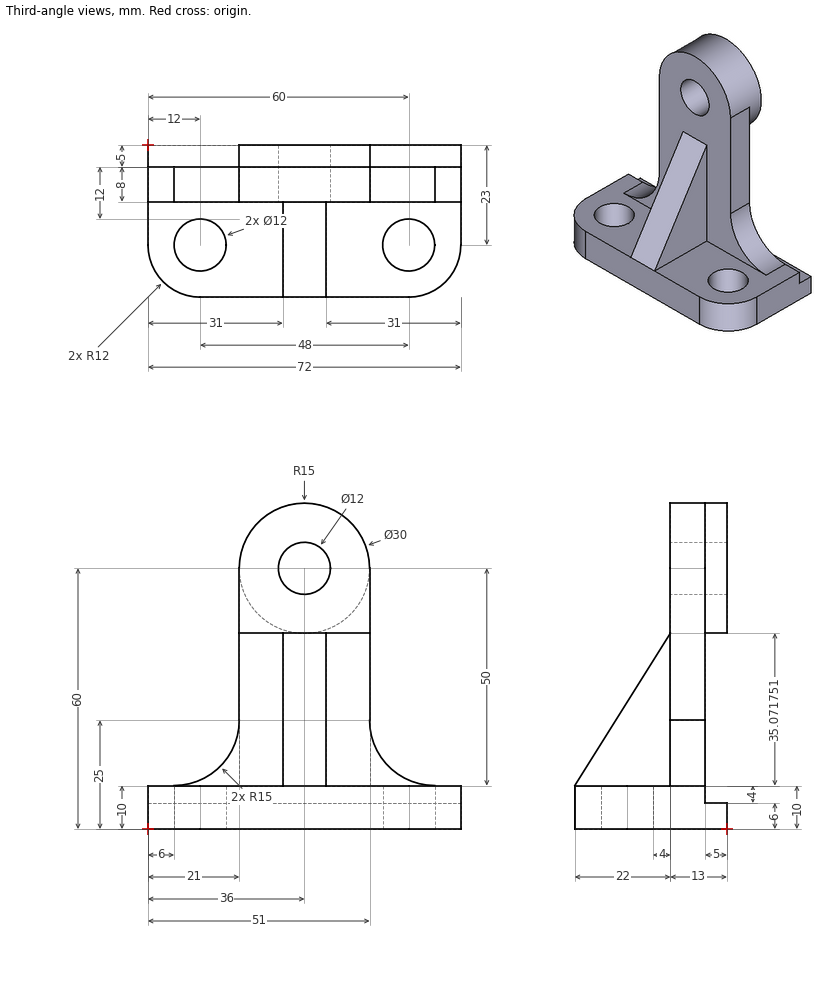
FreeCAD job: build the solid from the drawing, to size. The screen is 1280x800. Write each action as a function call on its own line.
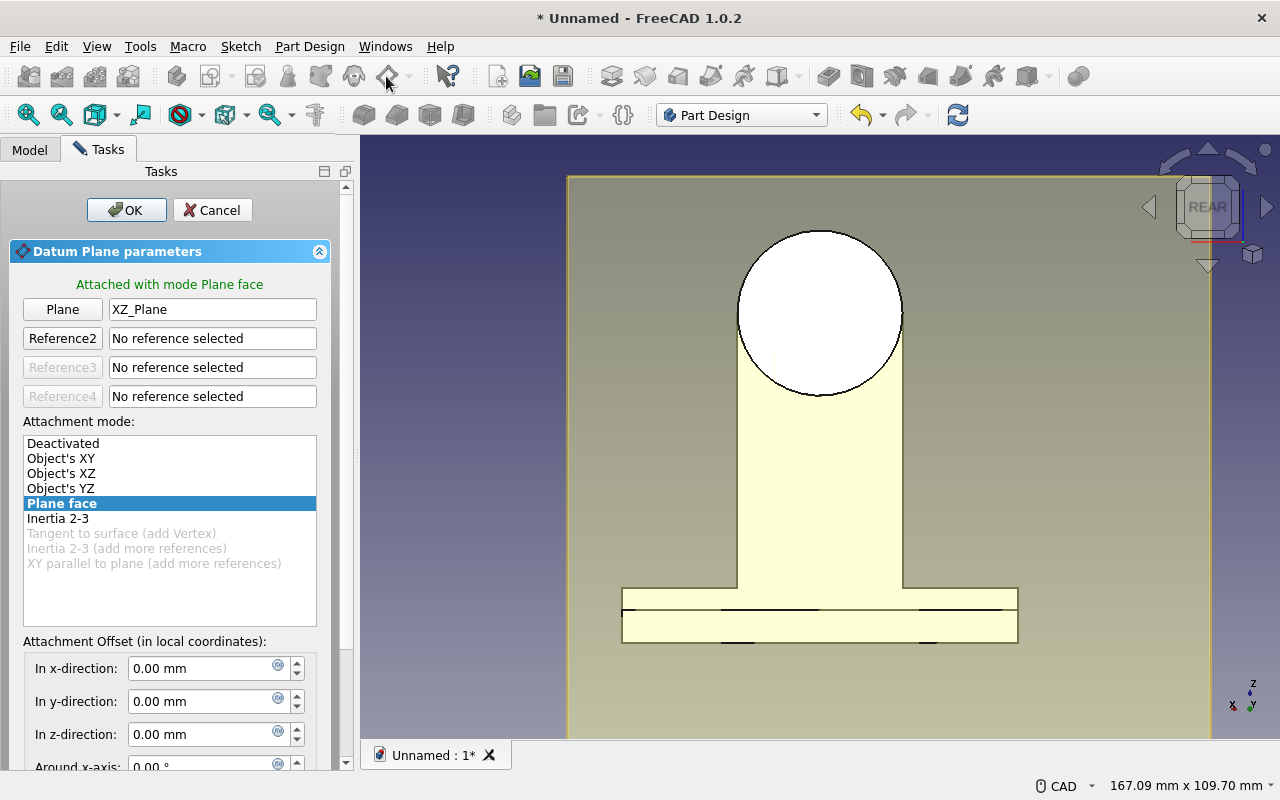
triple_click(210, 734)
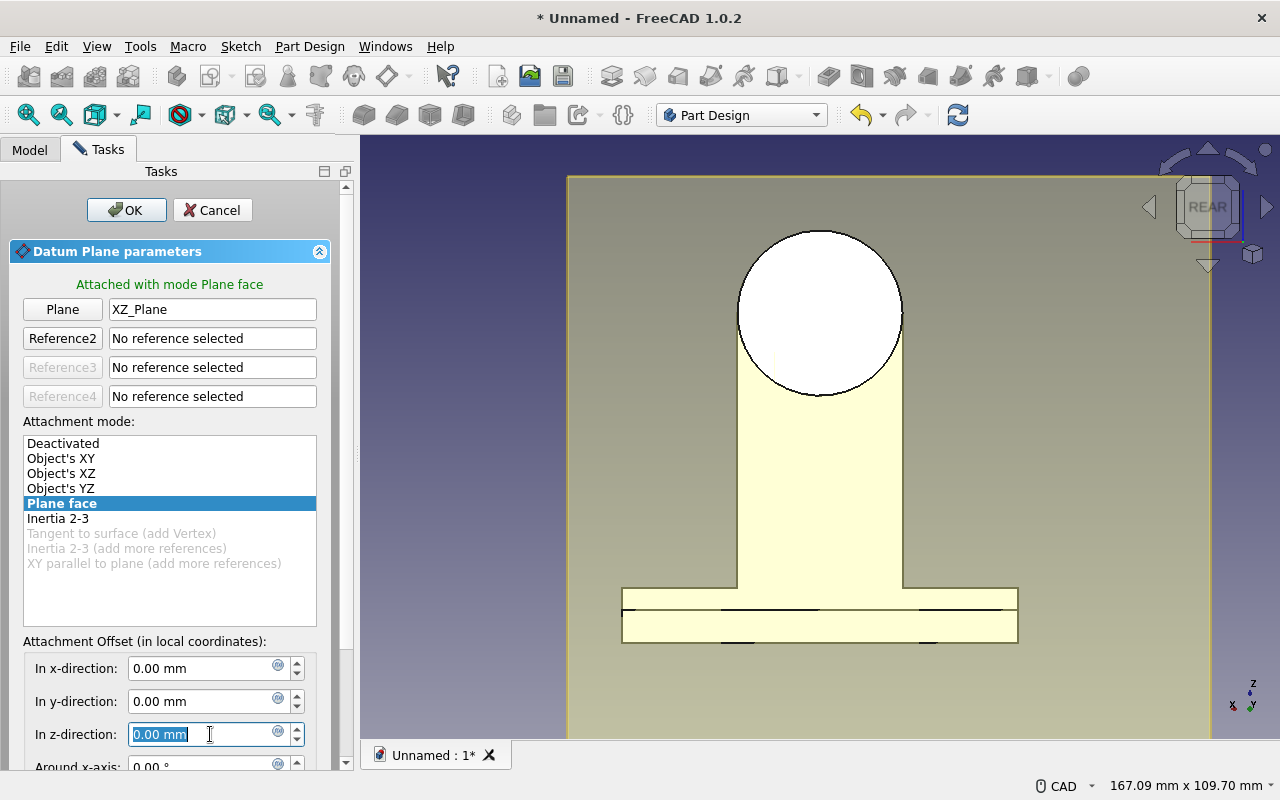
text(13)
key(Tab)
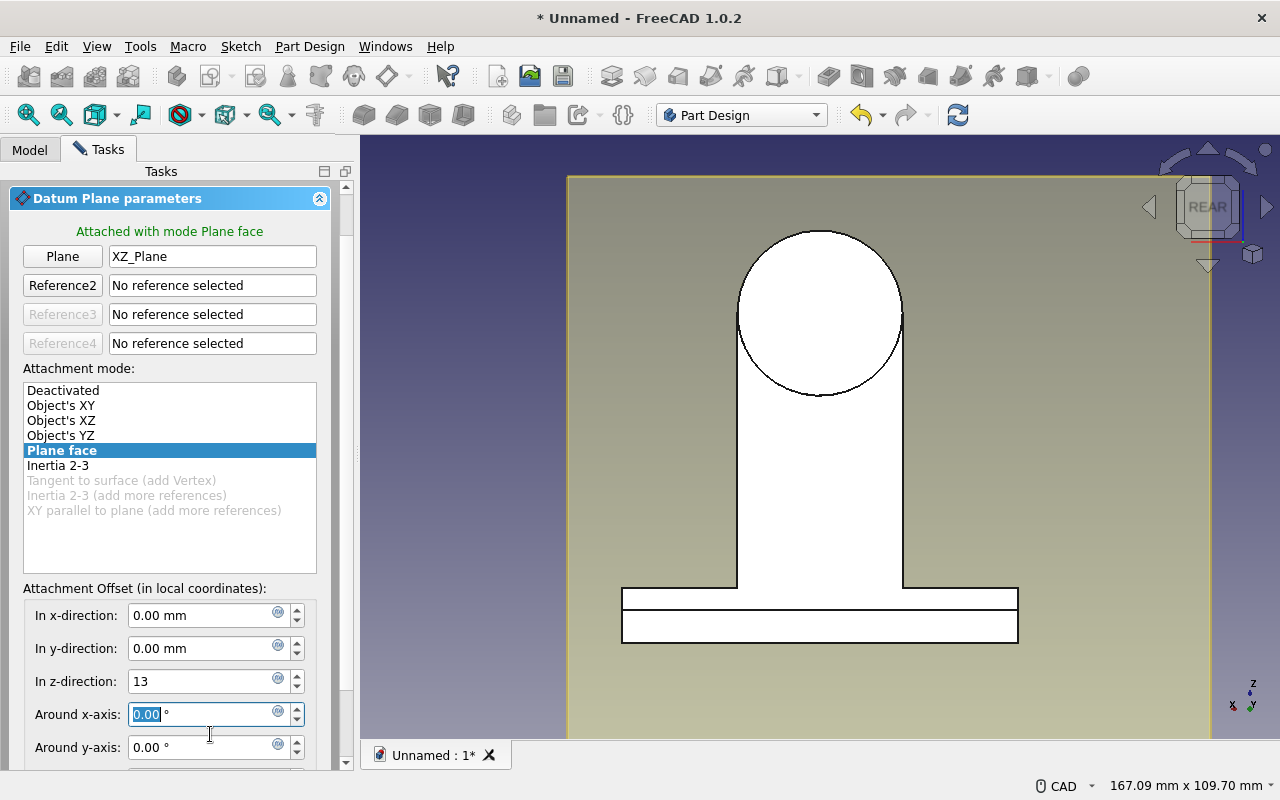
scroll(346, 476, up, 2)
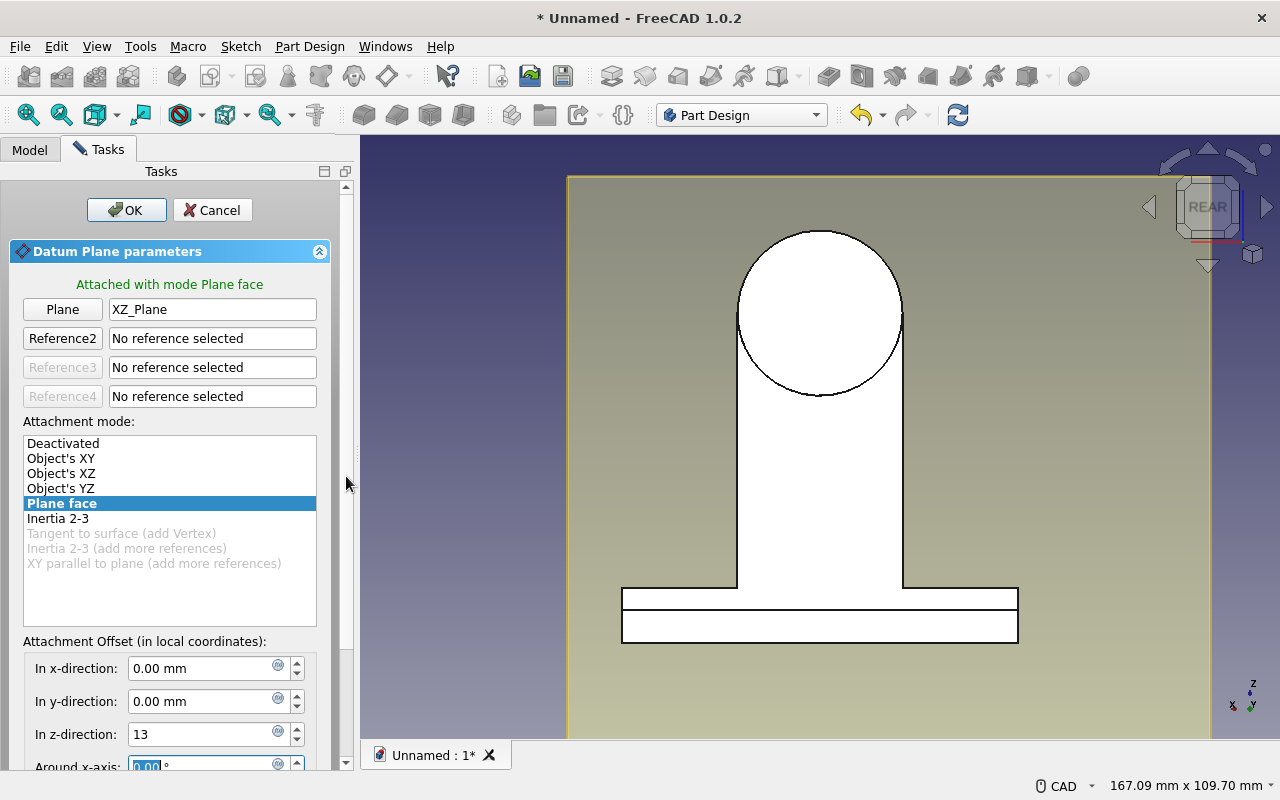
click(127, 210)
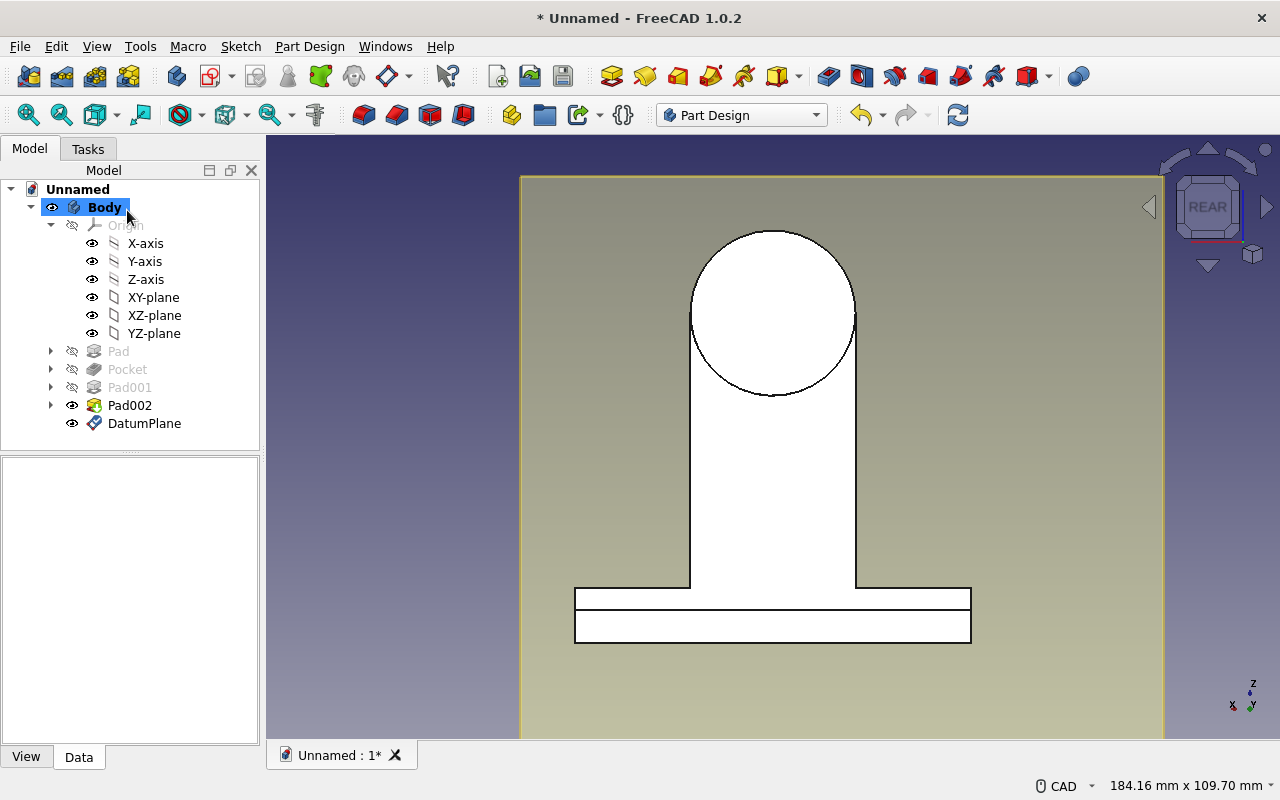
click(117, 423)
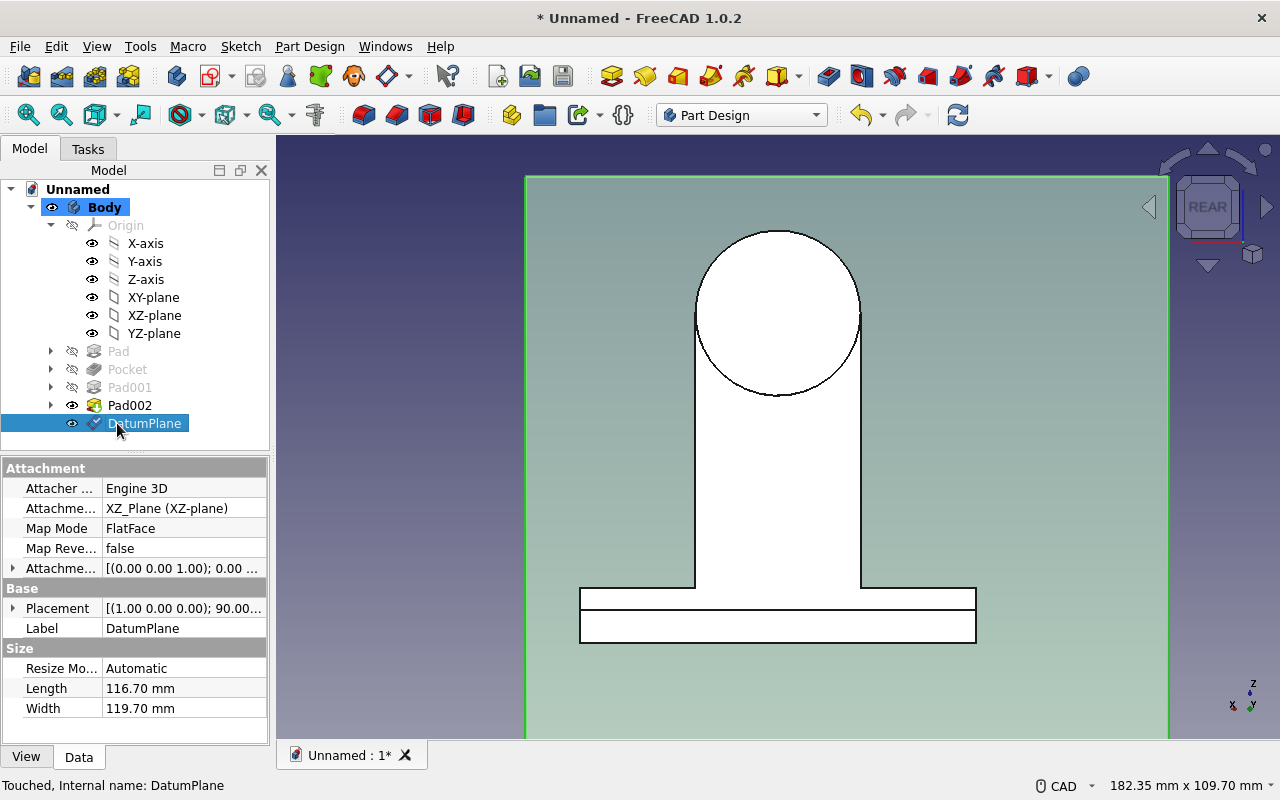
click(210, 76)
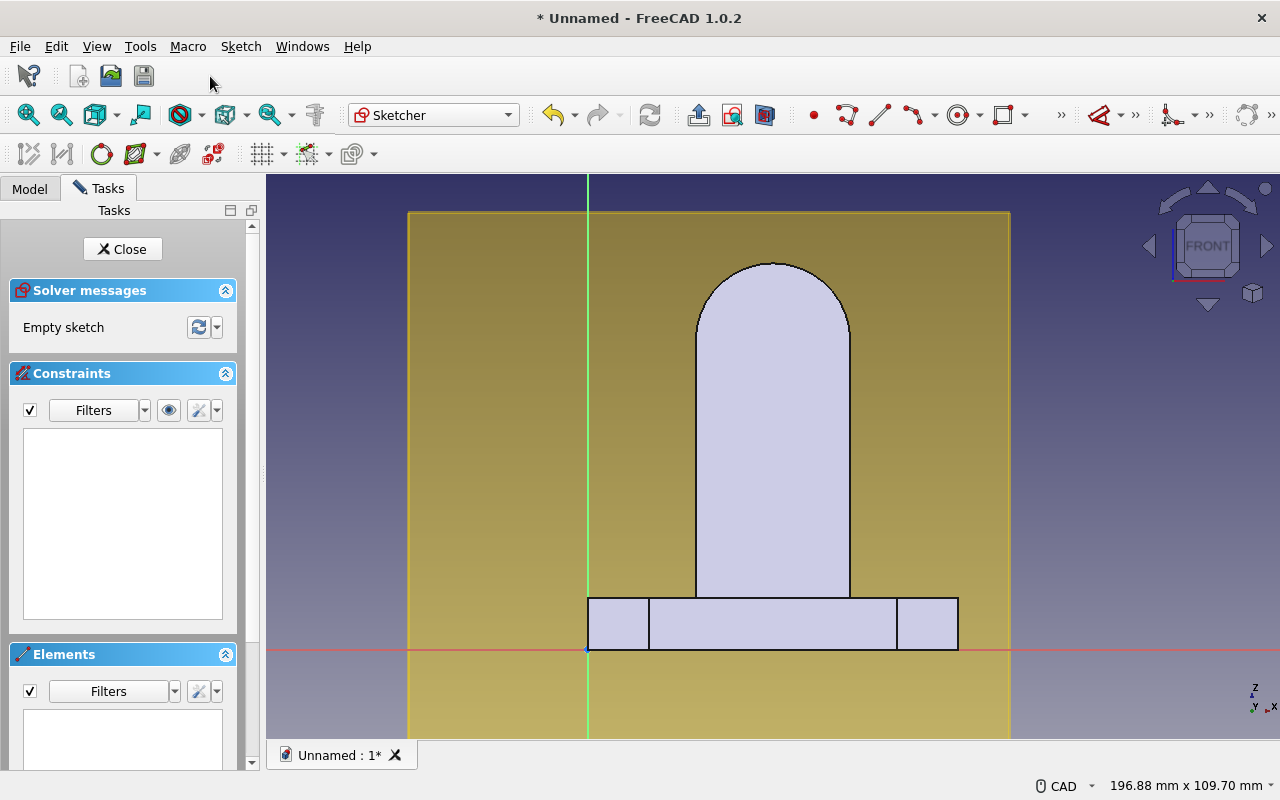
click(765, 116)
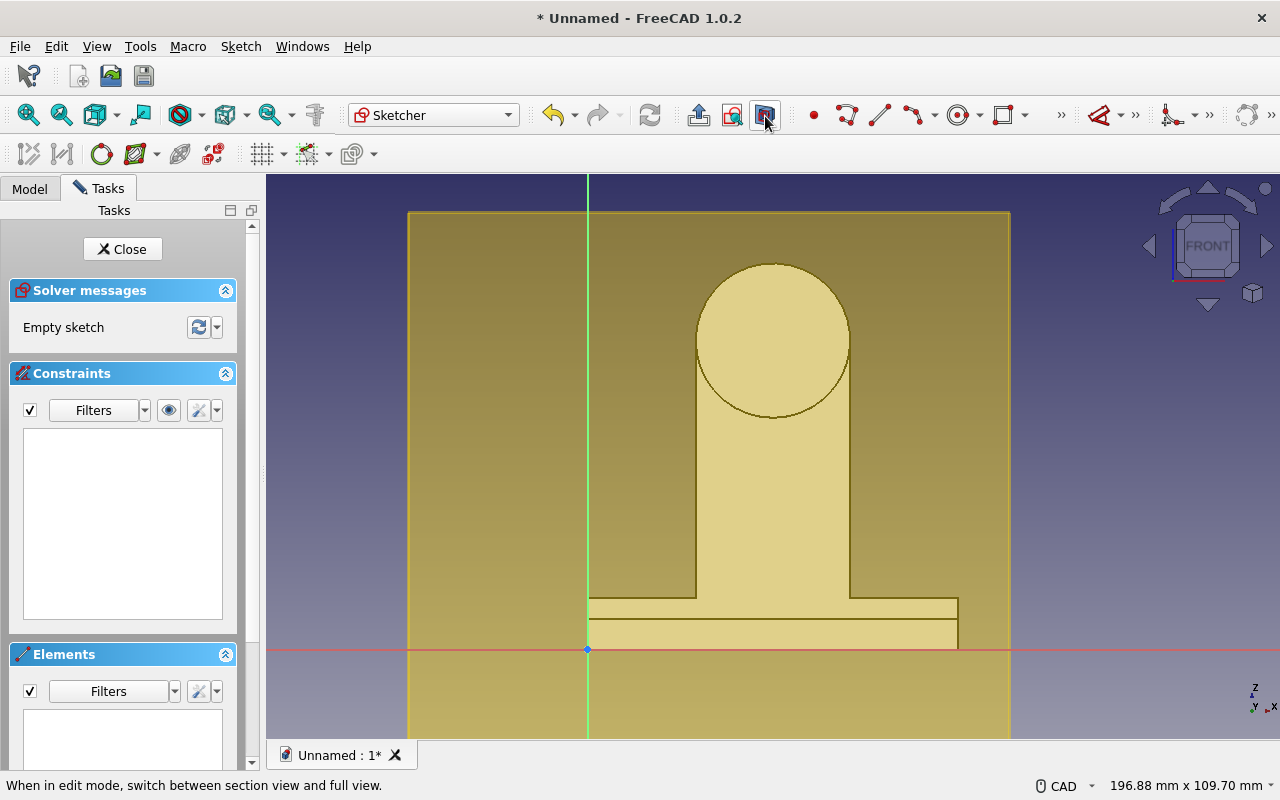
click(847, 116)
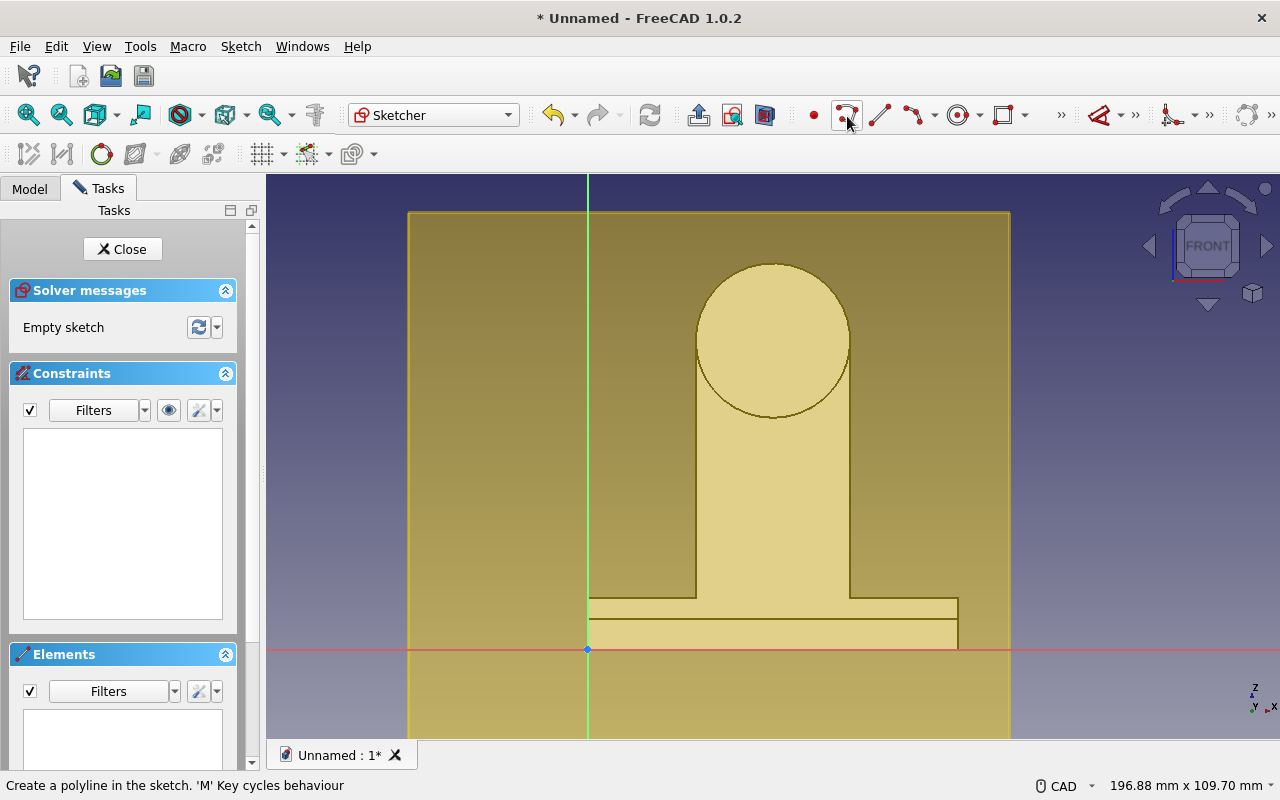
click(696, 341)
click(696, 598)
click(850, 598)
click(850, 341)
right_click(850, 341)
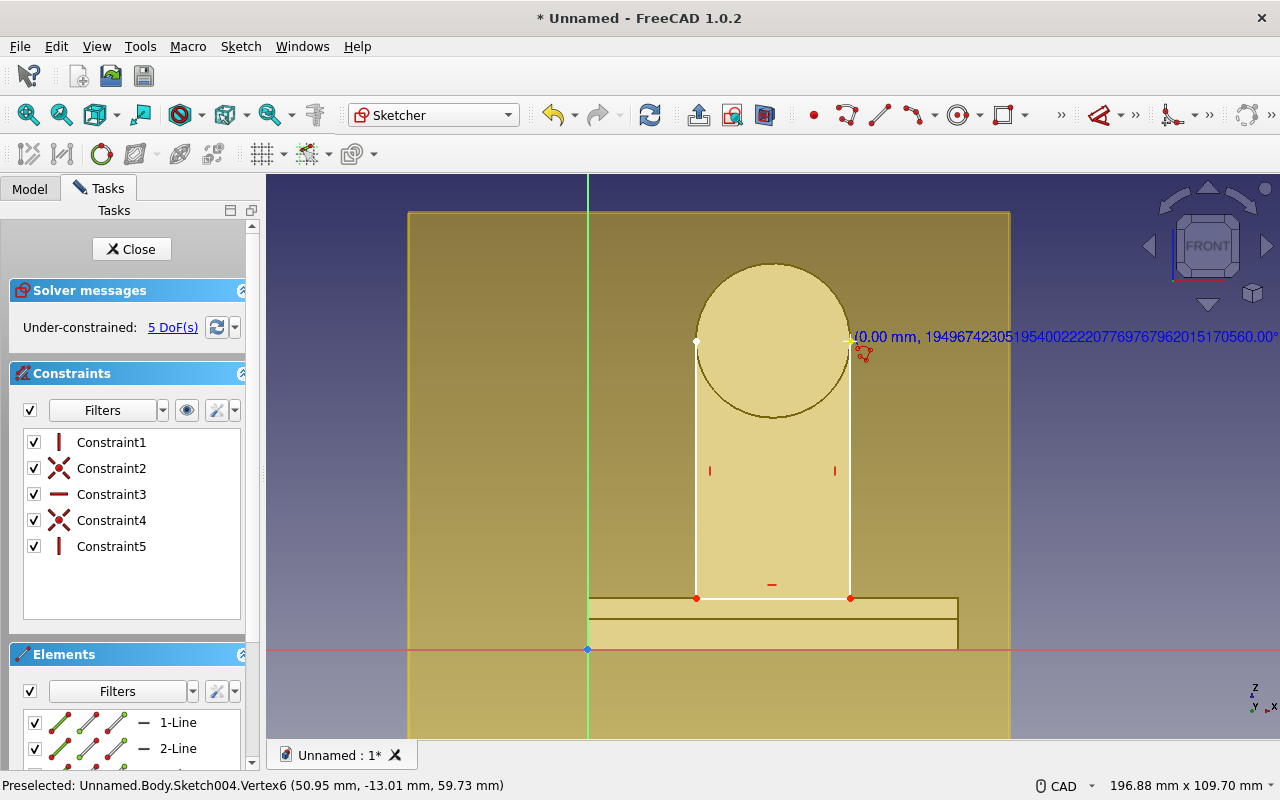
click(912, 116)